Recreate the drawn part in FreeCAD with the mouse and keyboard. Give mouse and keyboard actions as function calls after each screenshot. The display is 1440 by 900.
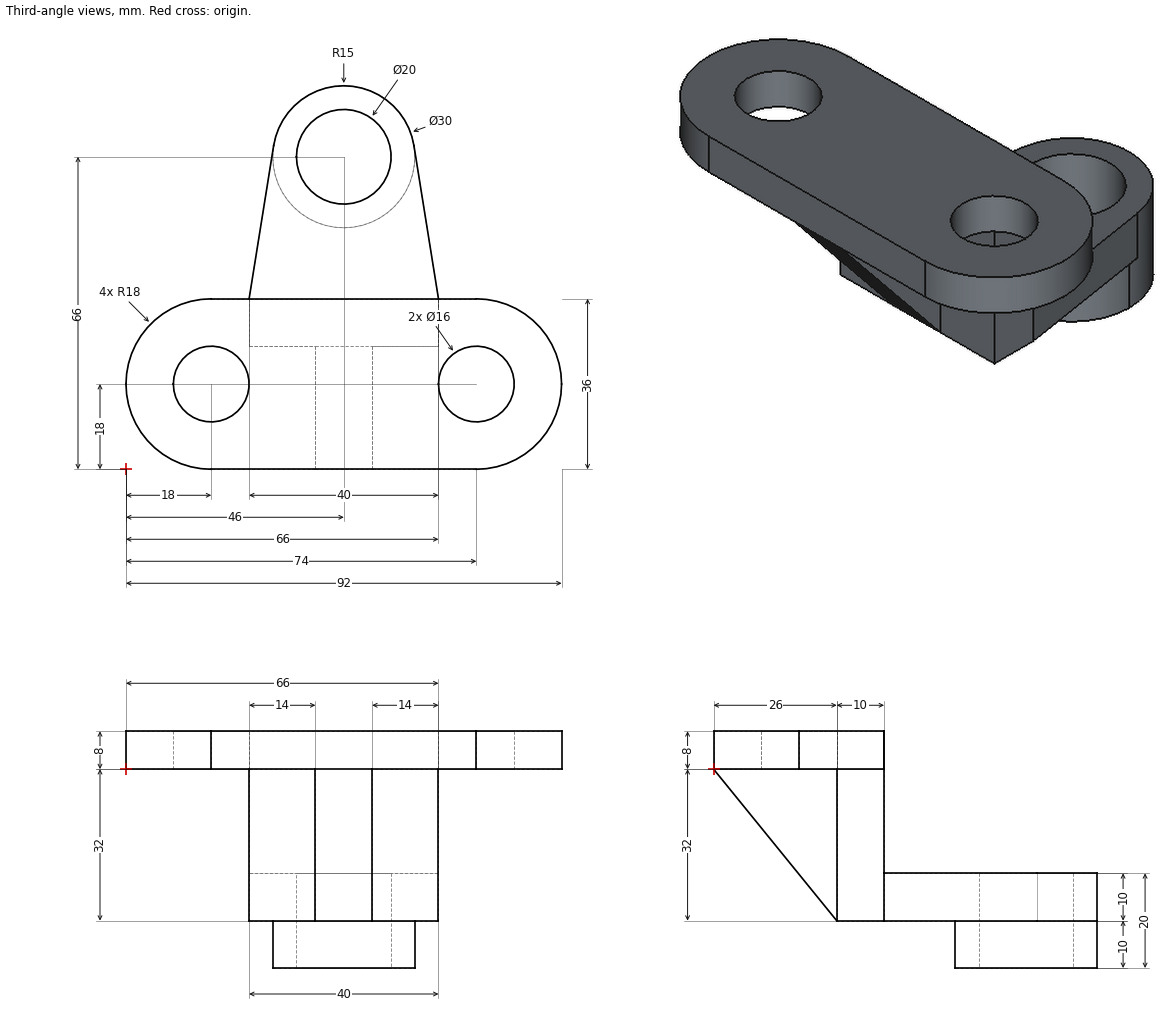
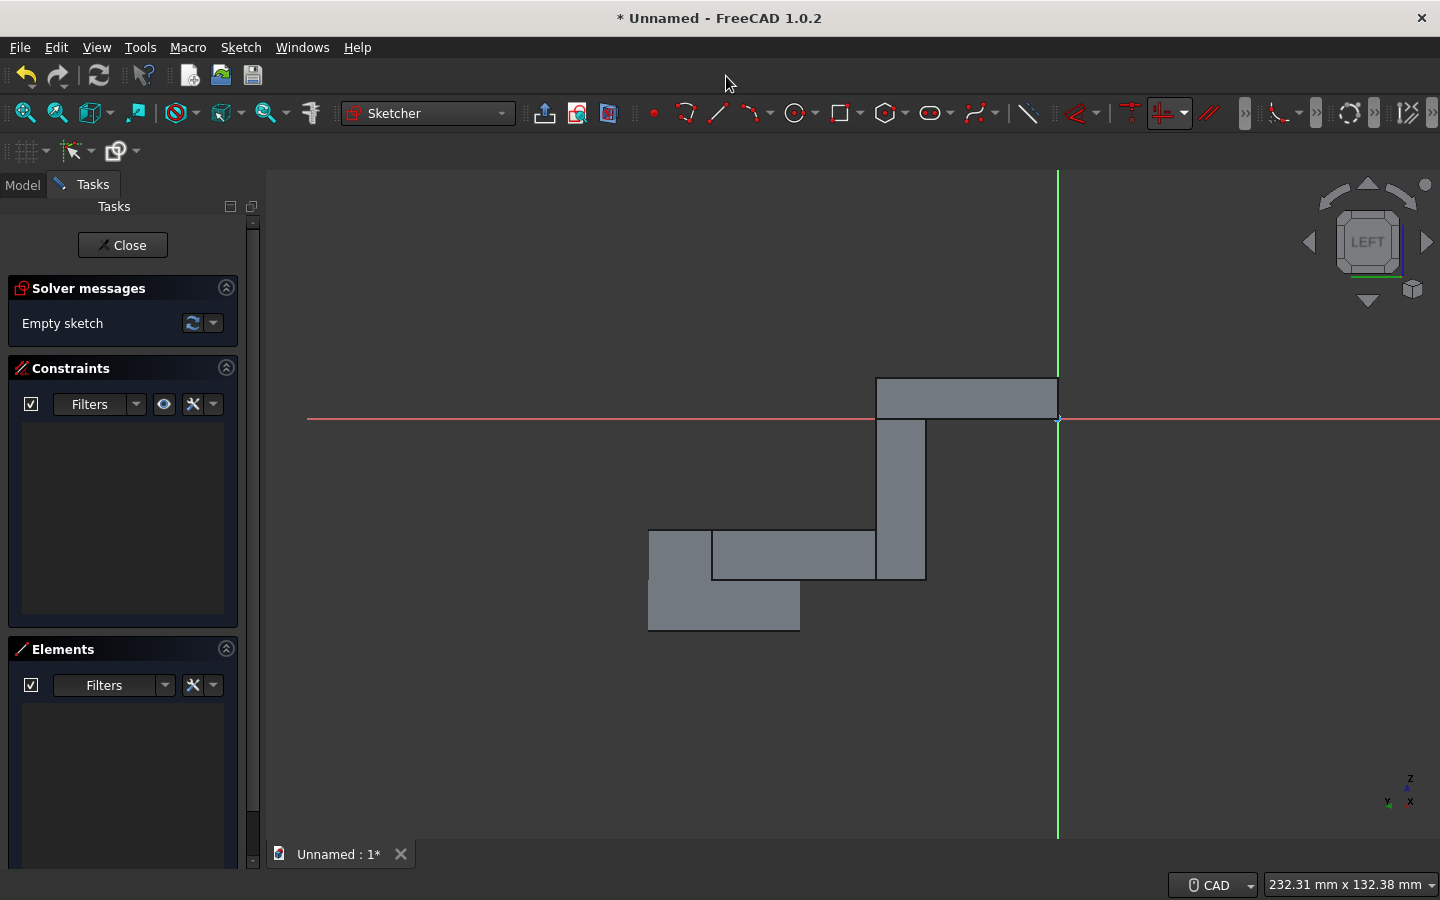
click(610, 114)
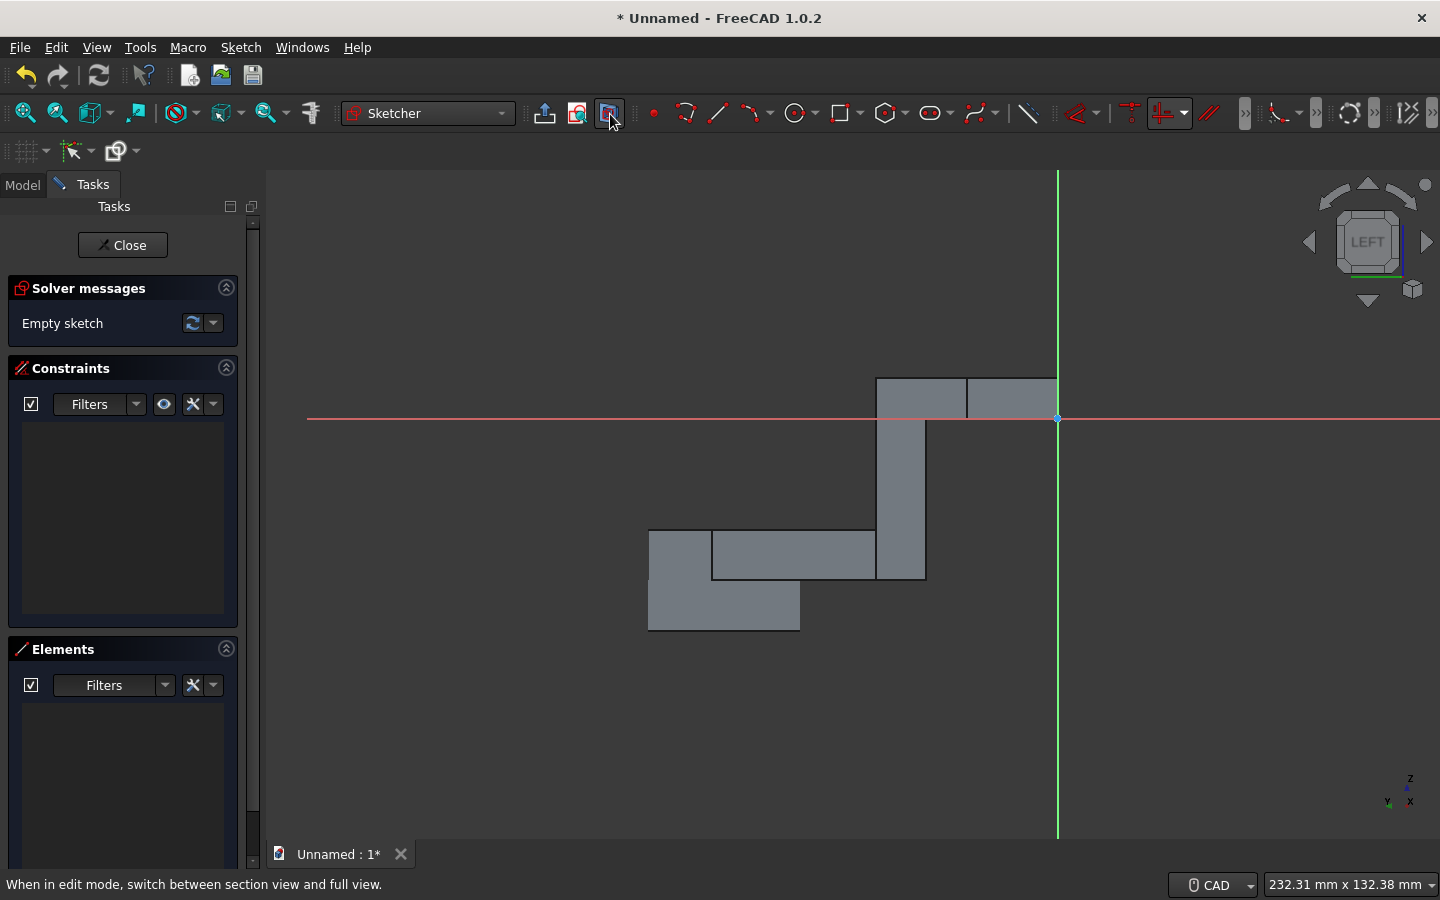
scroll(1113, 497, up, 5)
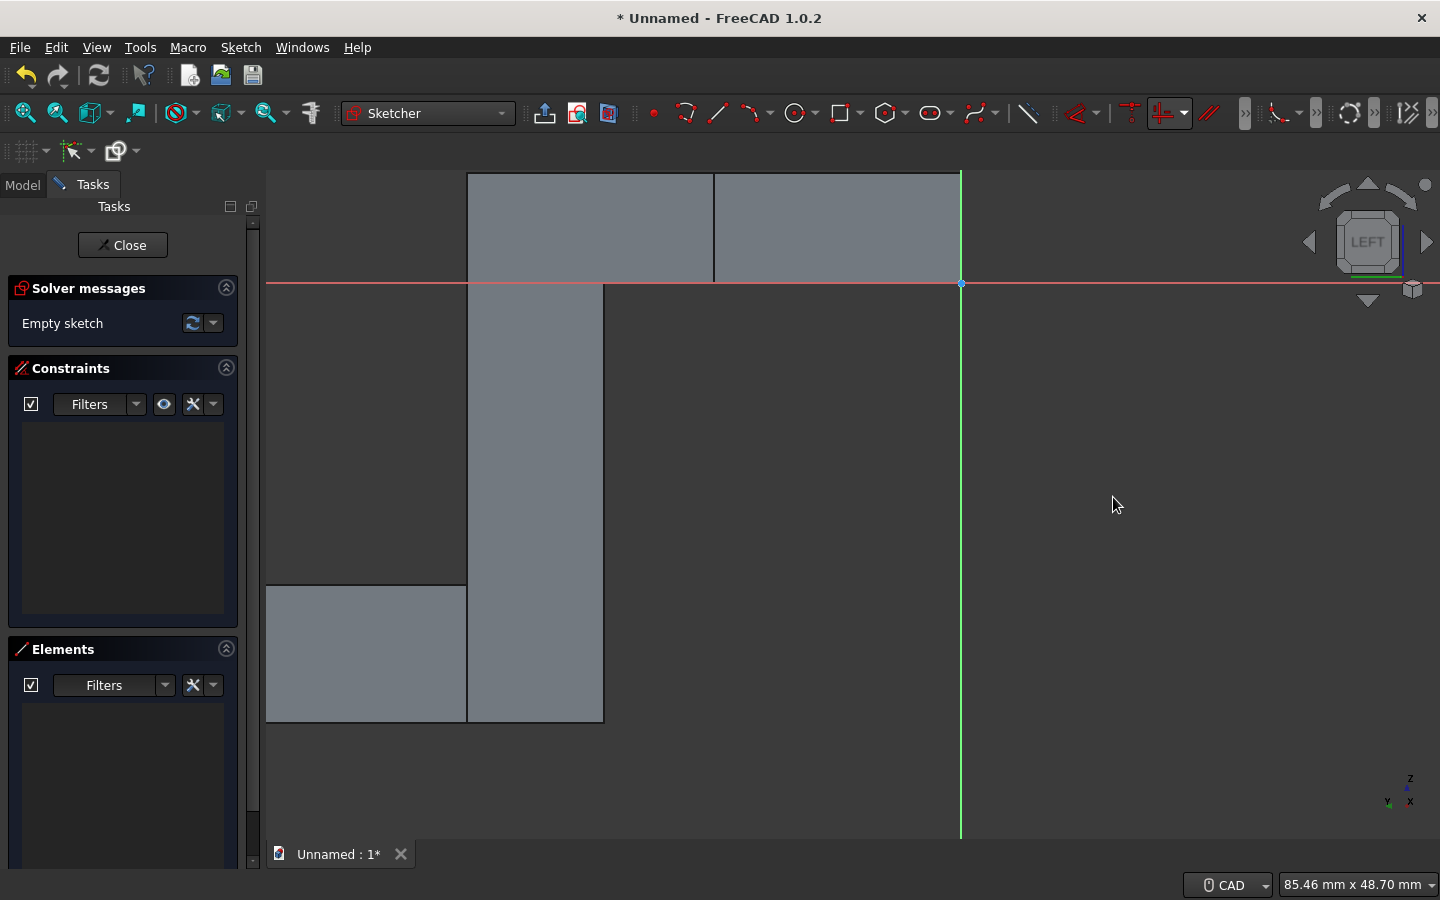
click(686, 114)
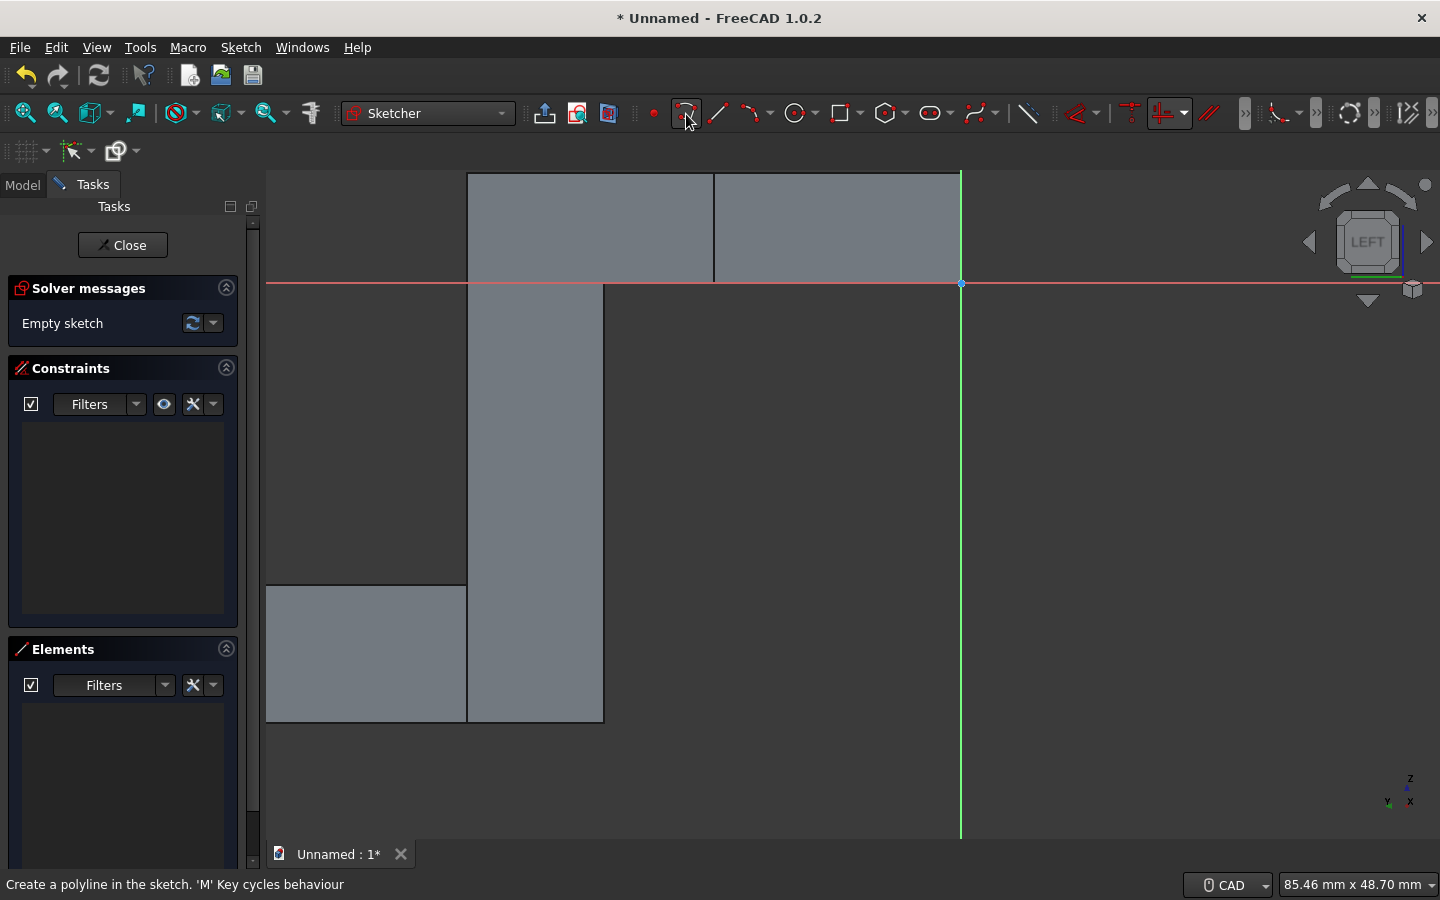
click(961, 283)
click(604, 292)
click(604, 723)
click(961, 283)
key(Escape)
key(Escape)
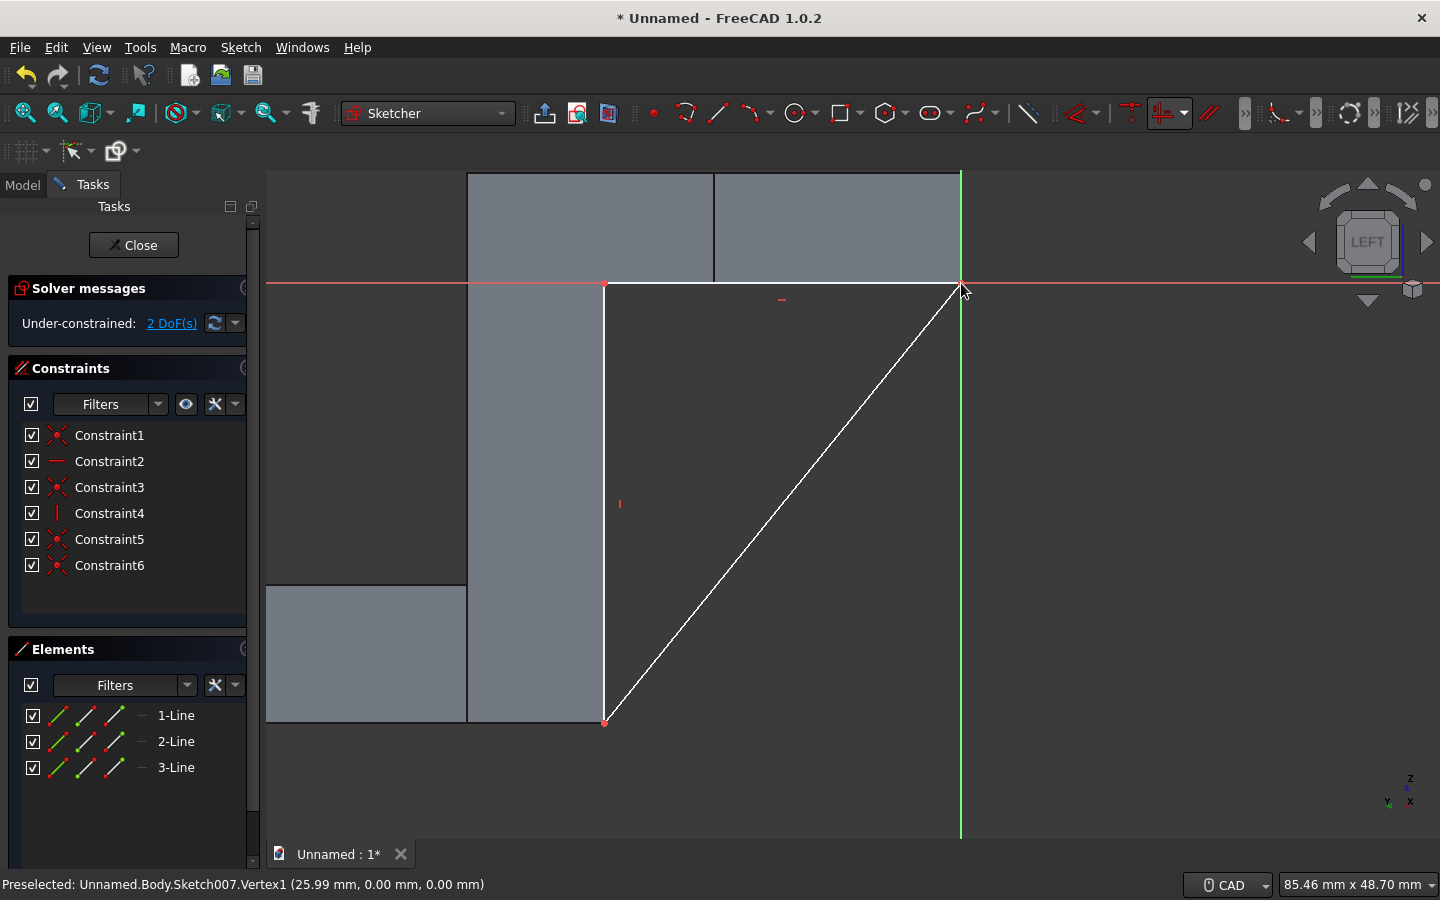
click(1076, 114)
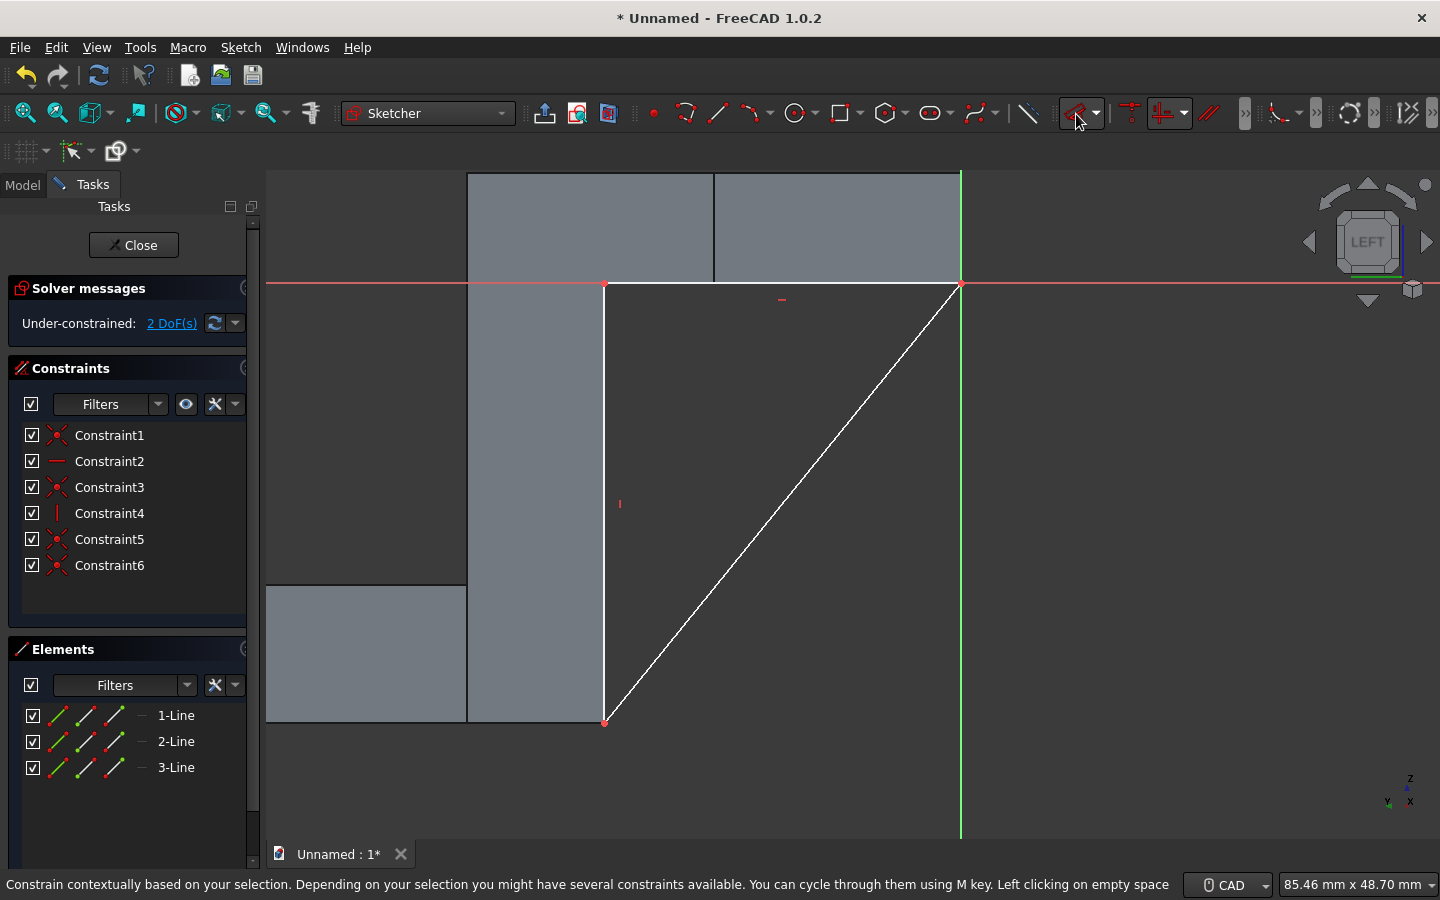
click(854, 283)
click(783, 249)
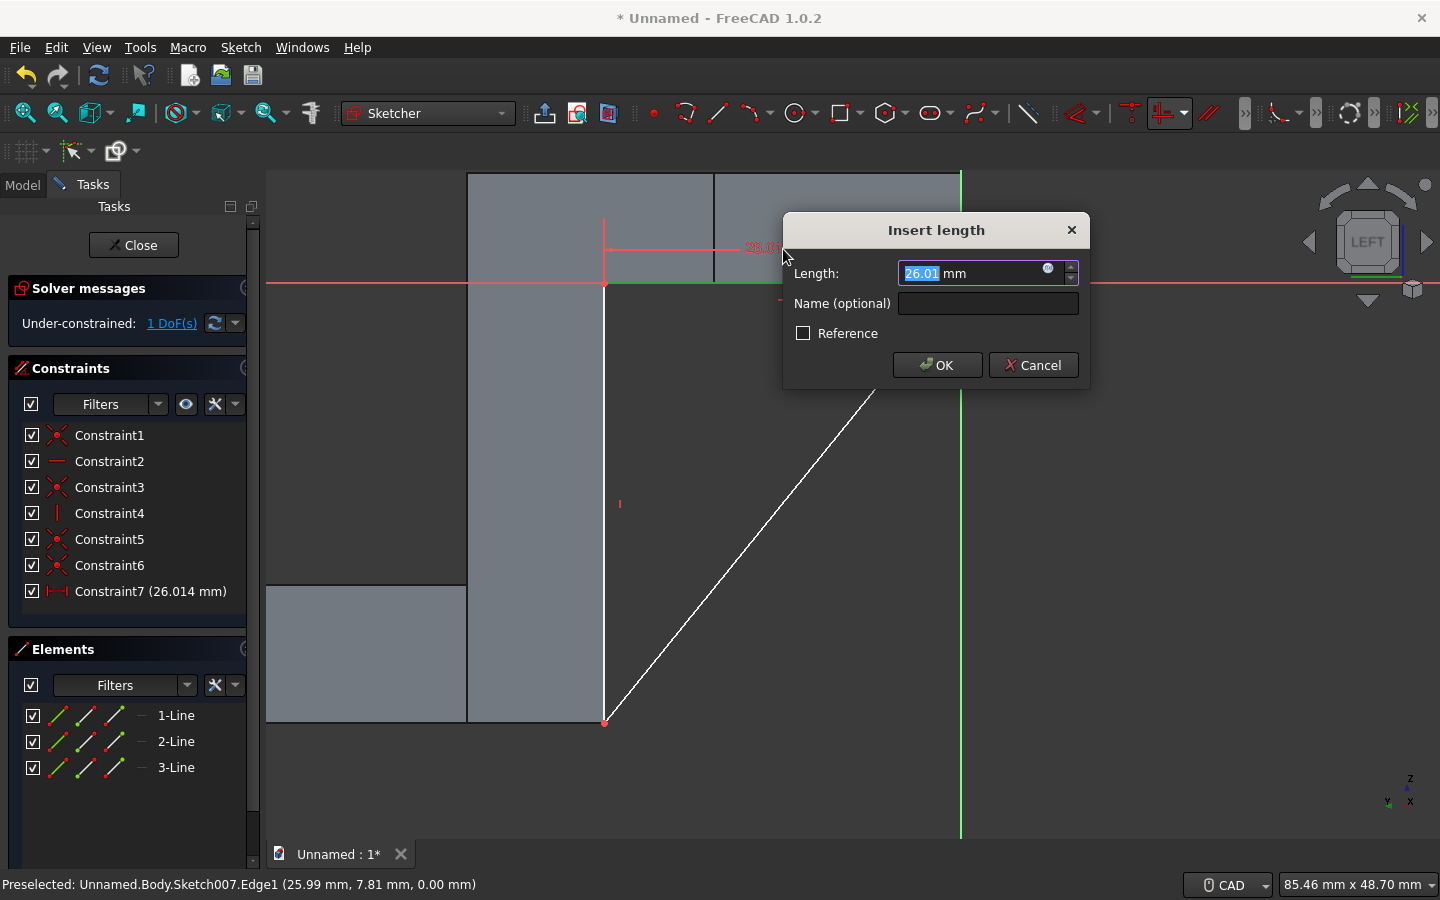
text(26)
key(Return)